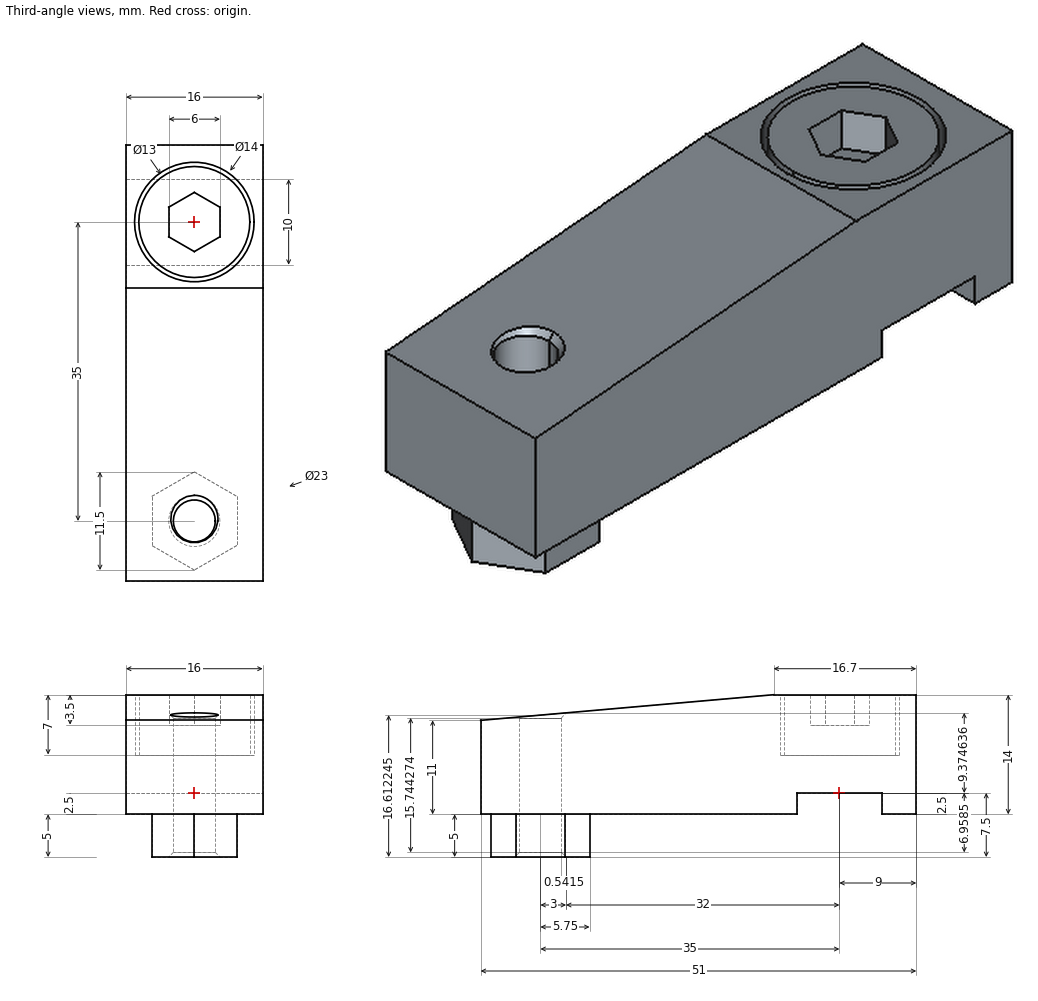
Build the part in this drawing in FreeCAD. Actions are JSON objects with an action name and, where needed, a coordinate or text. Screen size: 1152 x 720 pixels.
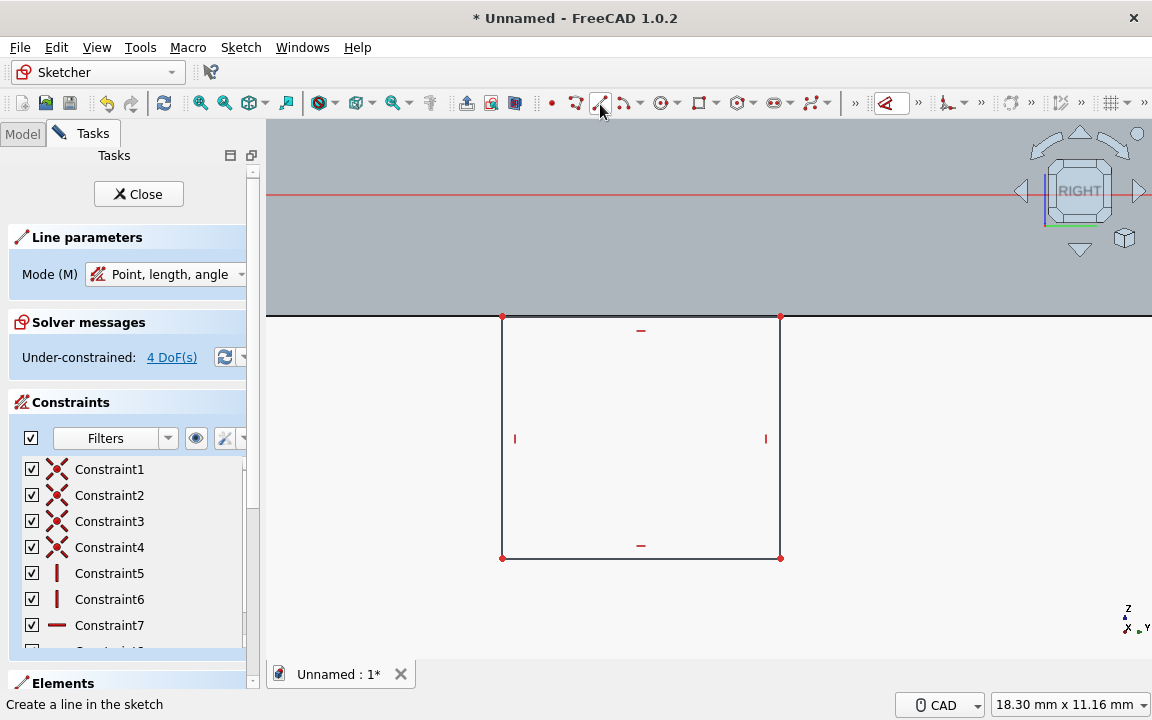
{"action": "left_click", "coordinate": [502, 291]}
{"action": "left_click", "coordinate": [502, 219]}
{"action": "key", "text": "Escape"}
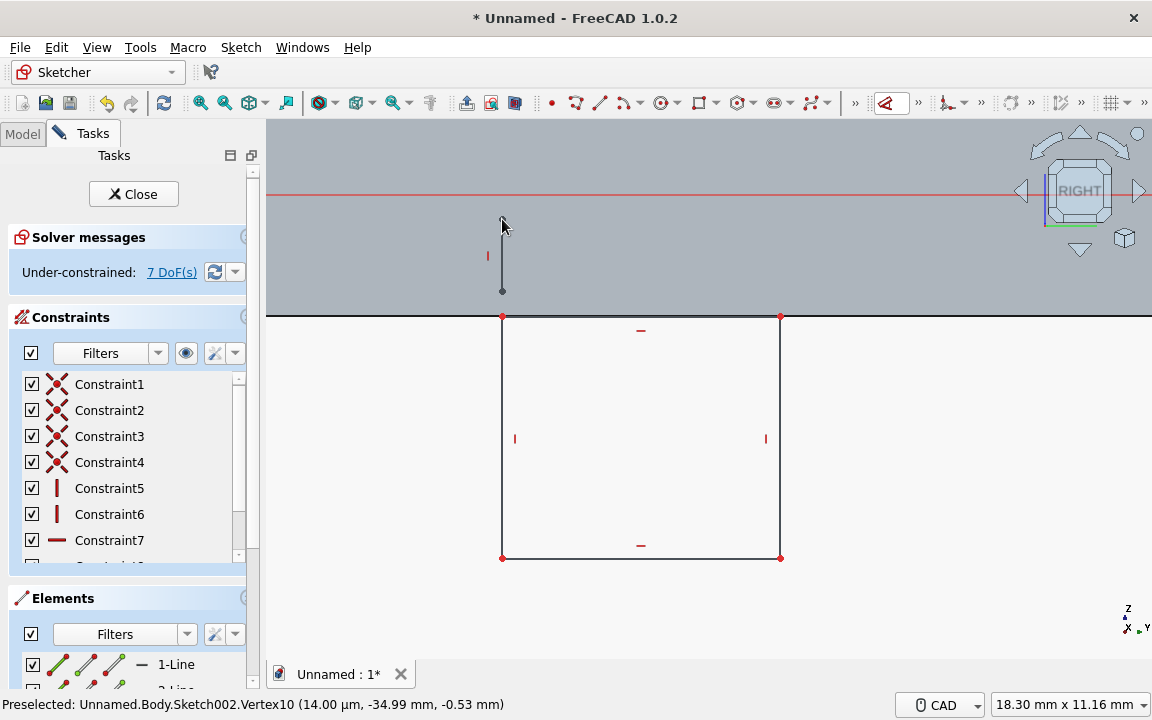
{"action": "left_click", "coordinate": [502, 270]}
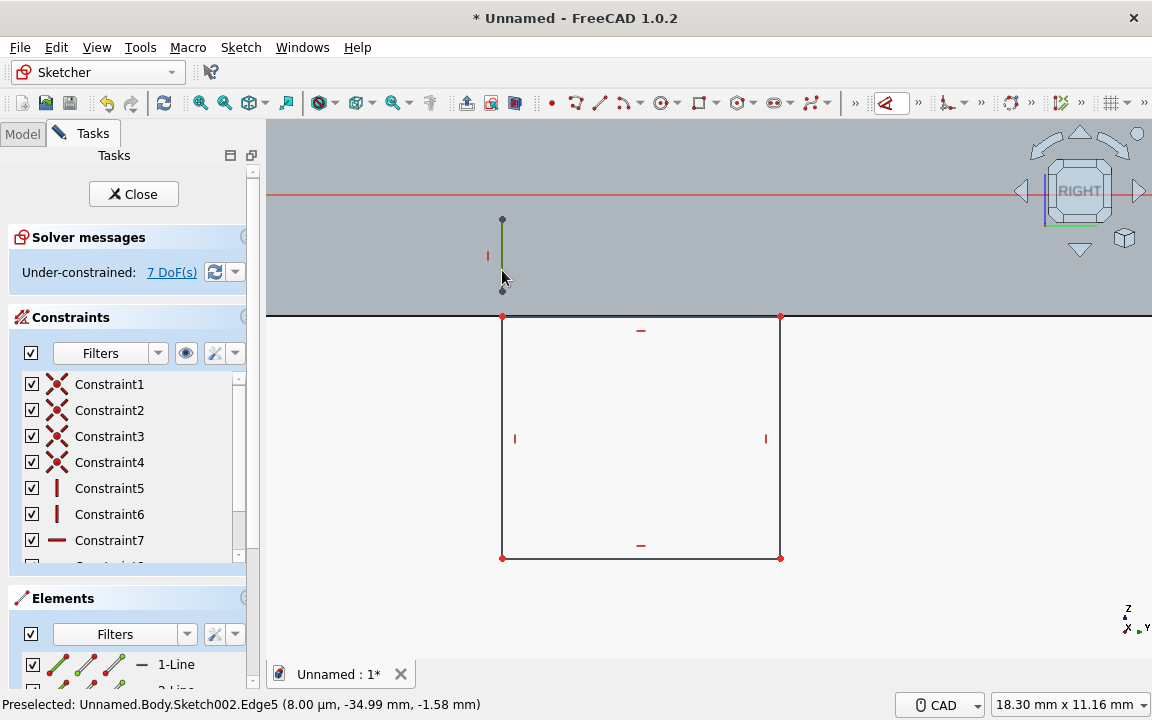
{"action": "key", "text": "g n"}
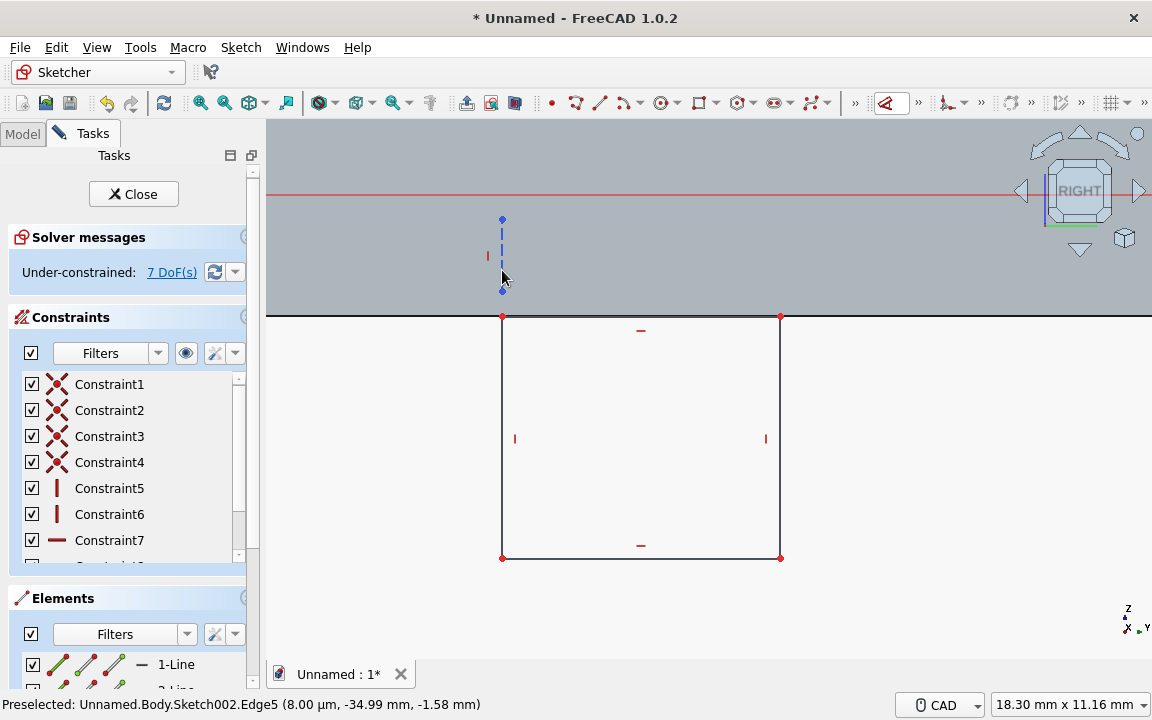
{"action": "left_click", "coordinate": [502, 390]}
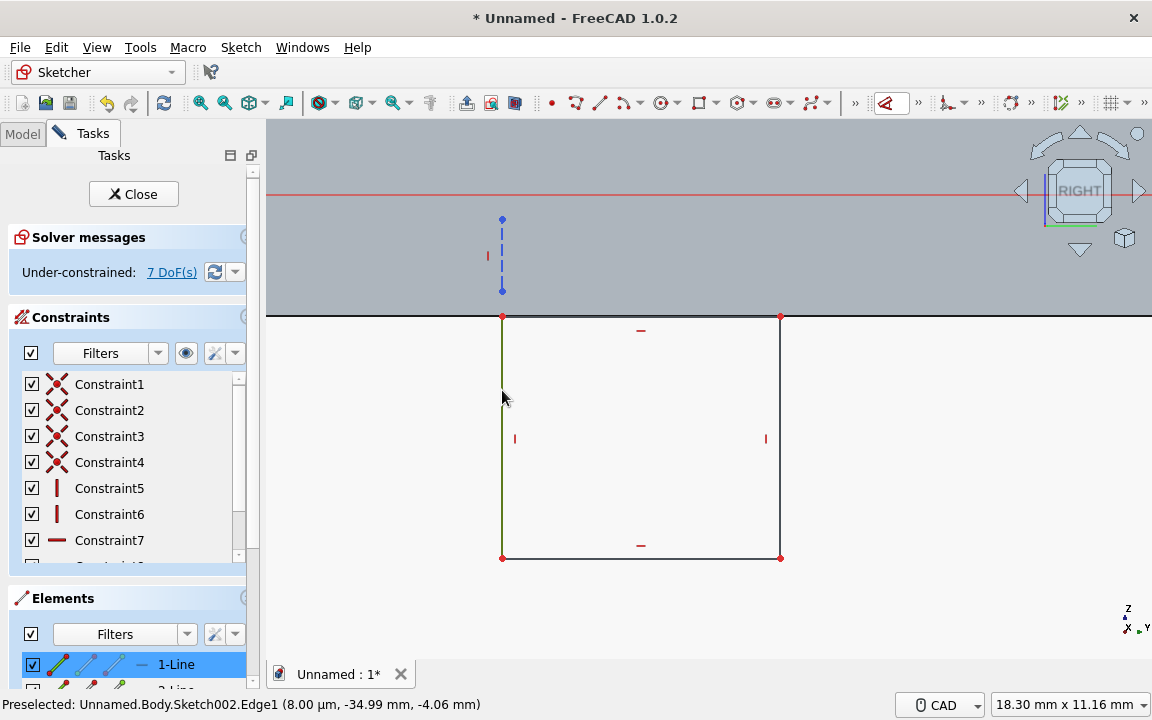
{"action": "left_click", "coordinate": [904, 104]}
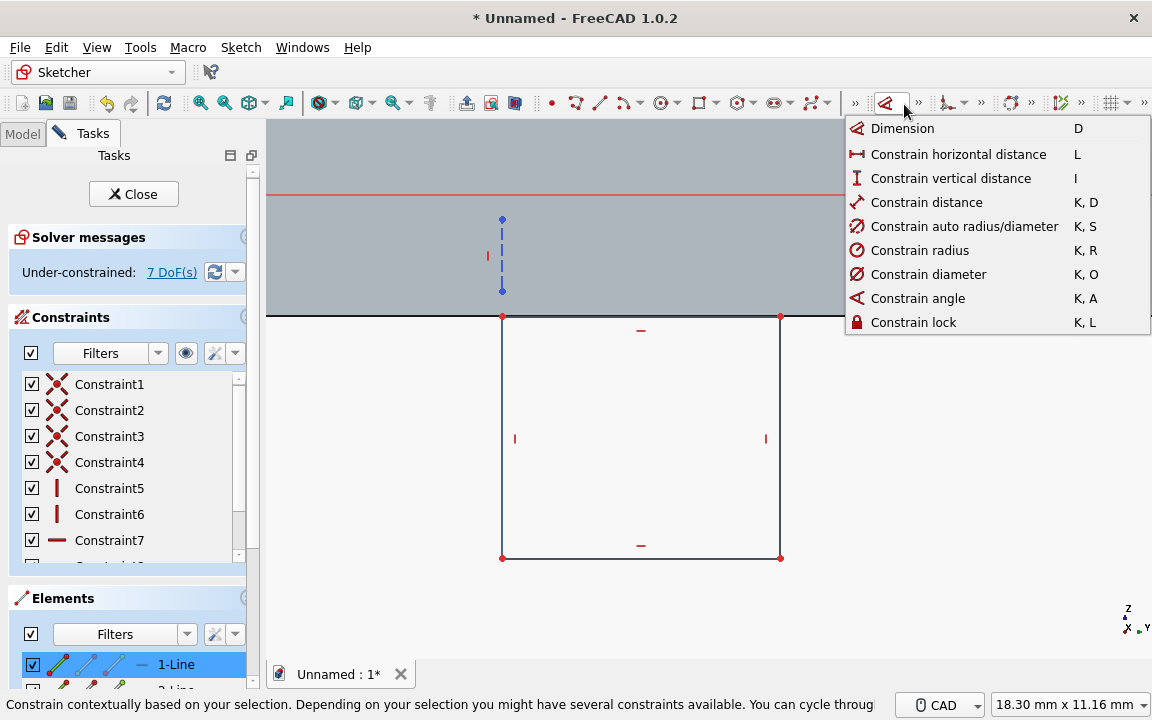
{"action": "left_click", "coordinate": [998, 178]}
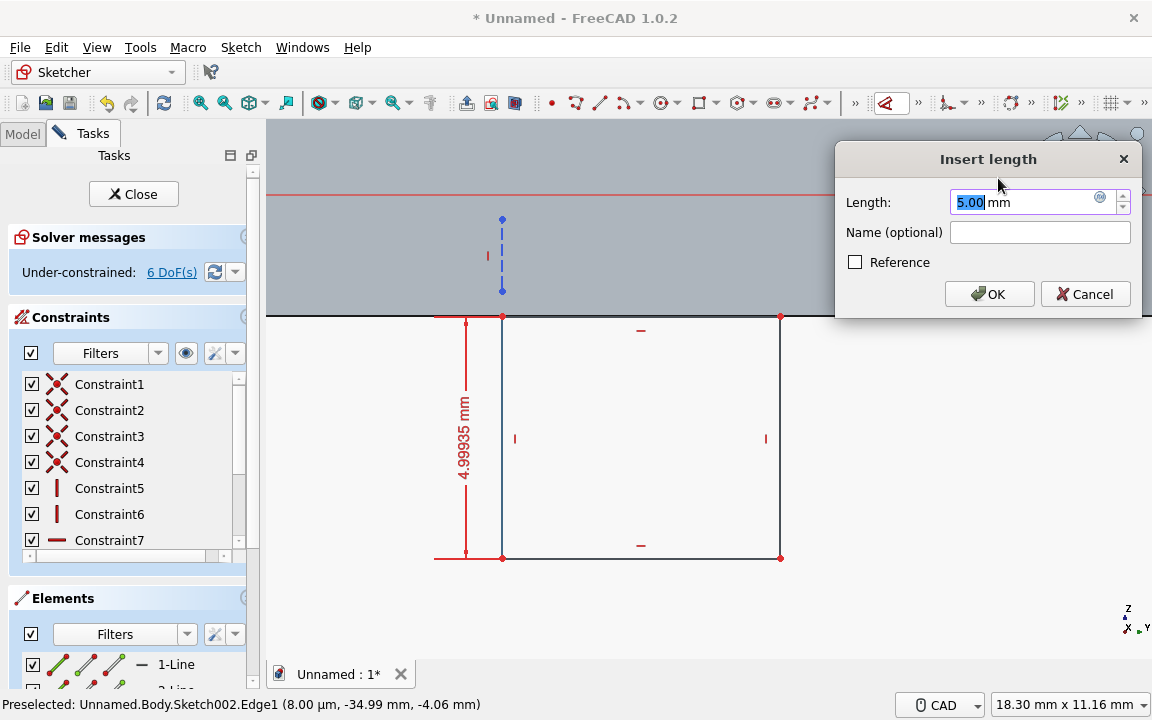
{"action": "type", "text": "5"}
{"action": "key", "text": "Return"}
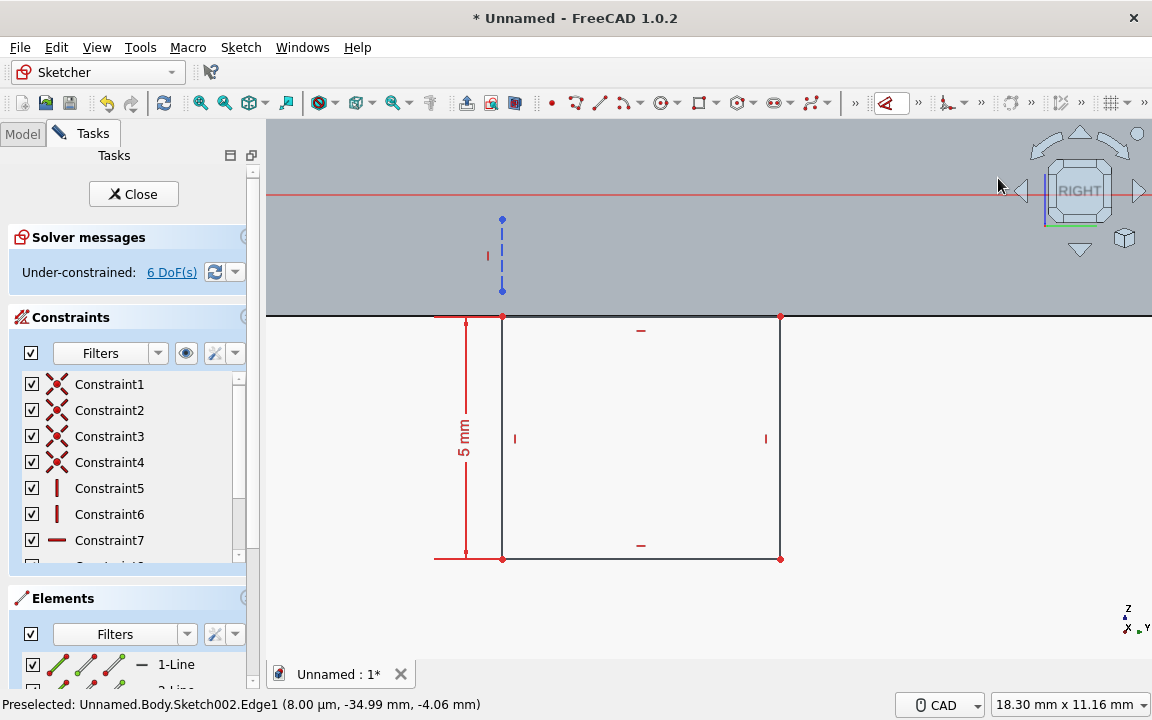
{"action": "left_click", "coordinate": [502, 317]}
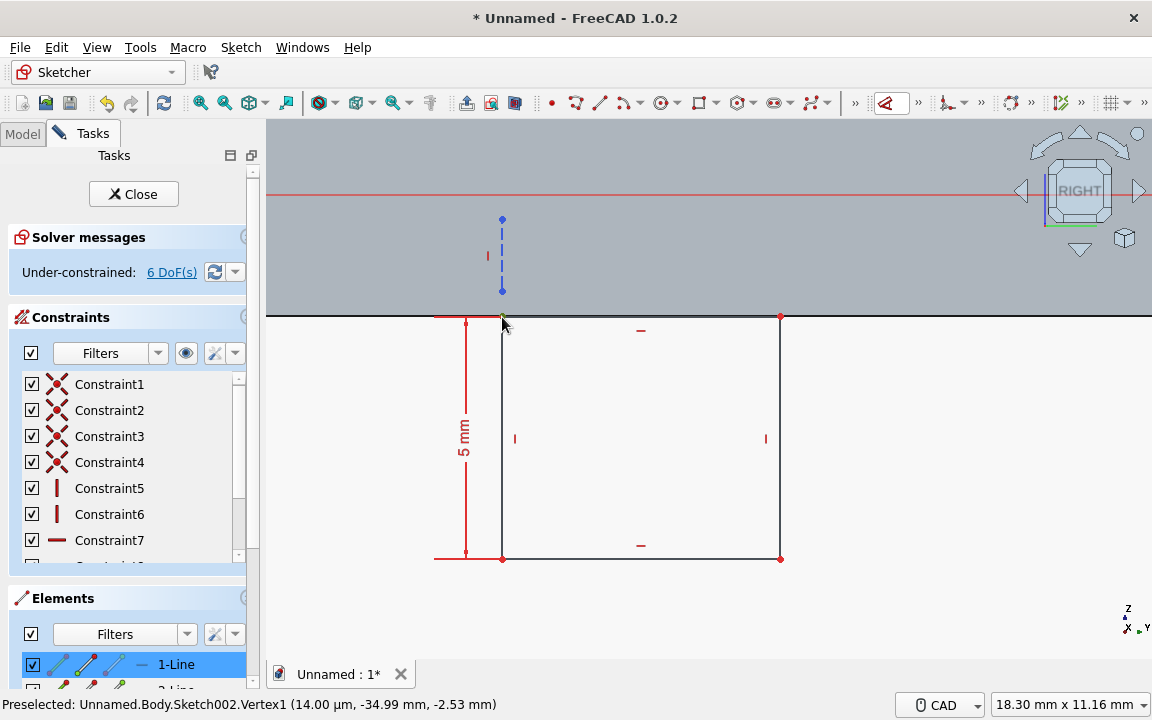
{"action": "key", "text": "l"}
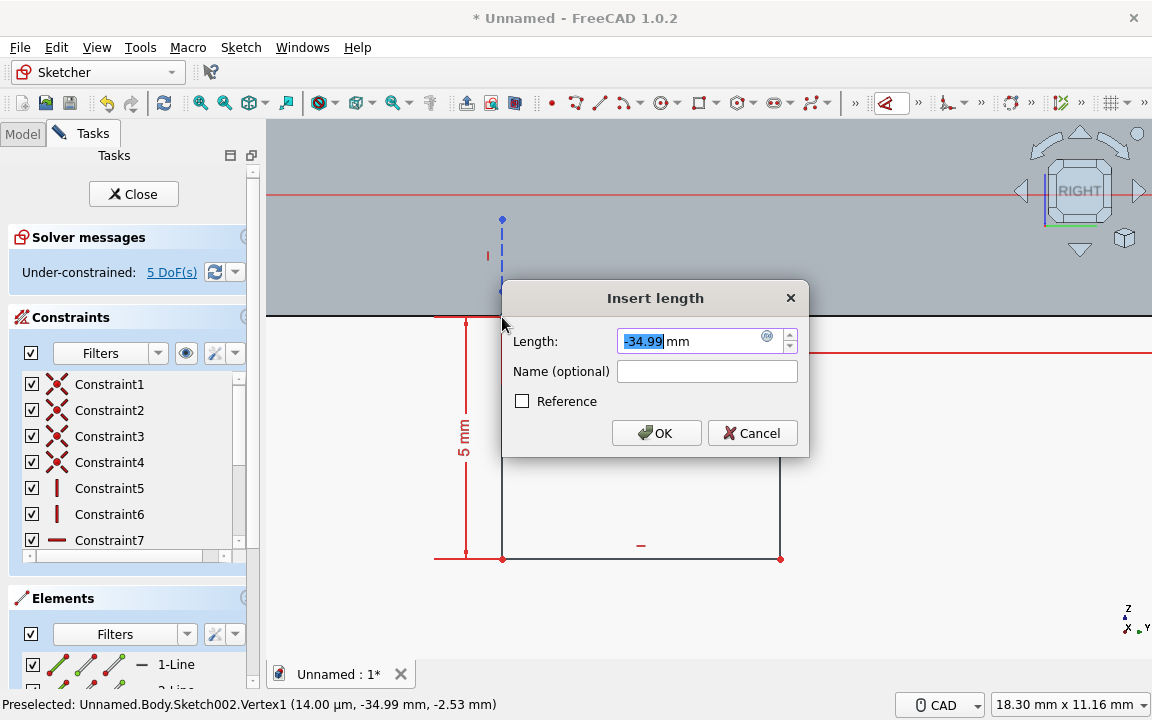
{"action": "type", "text": "-35"}
{"action": "key", "text": "Return"}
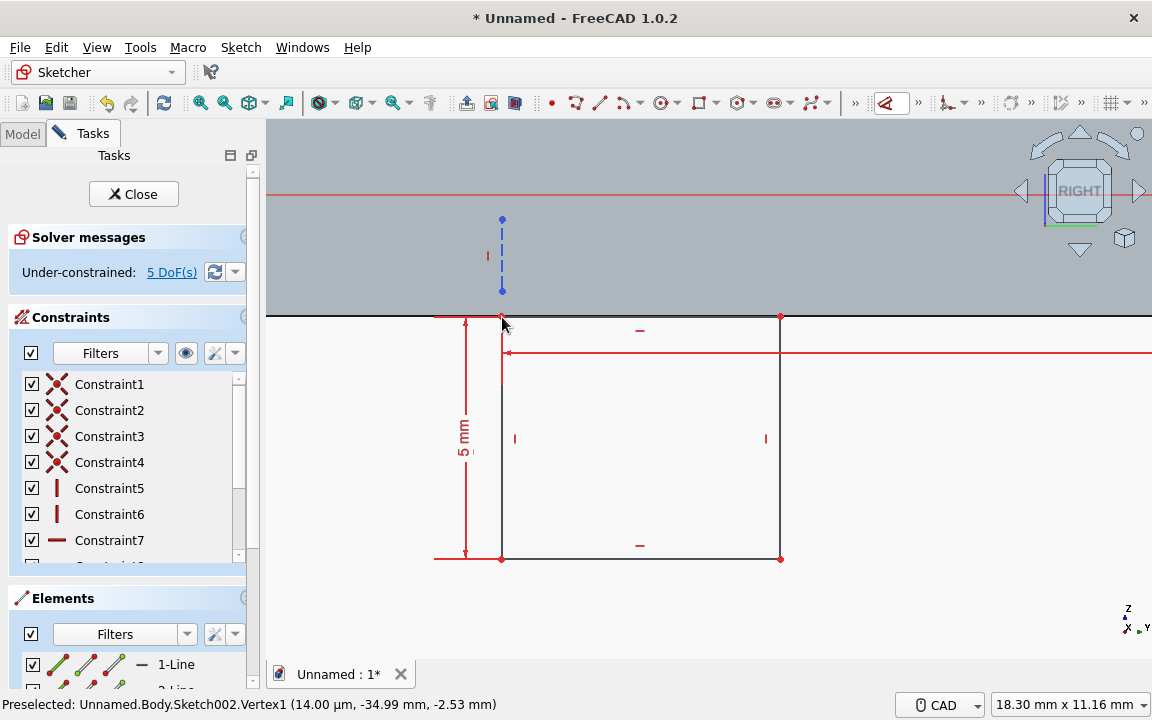
{"action": "left_click", "coordinate": [502, 292]}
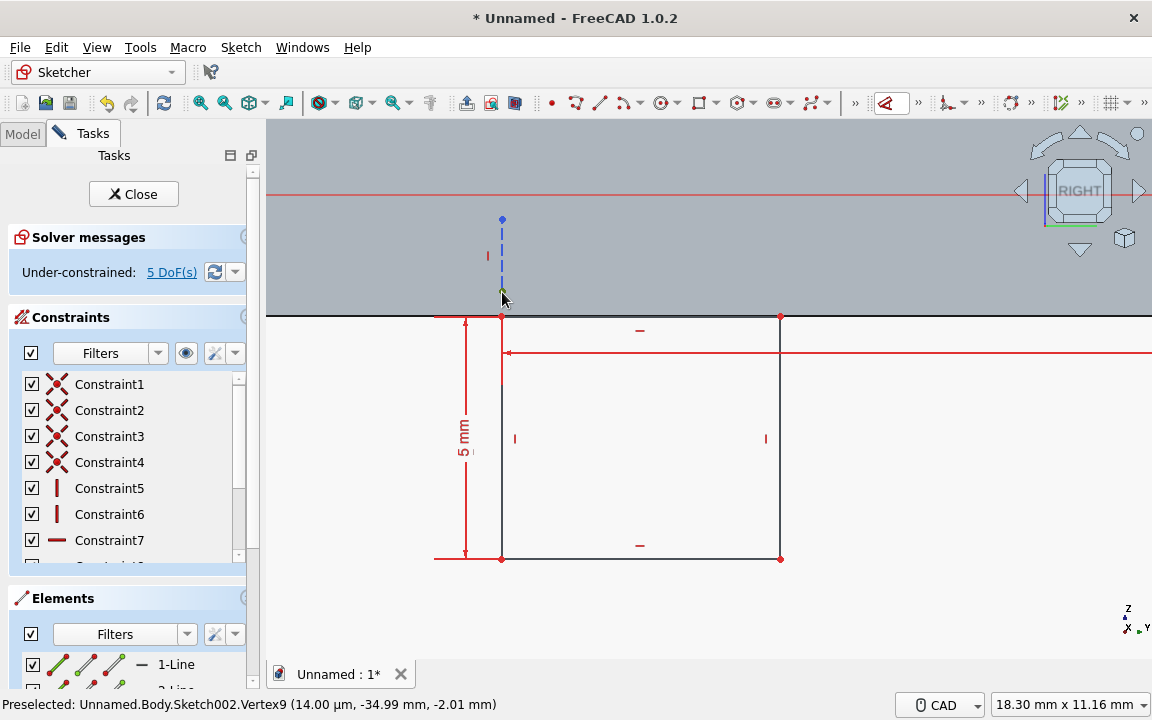
{"action": "key", "text": "l"}